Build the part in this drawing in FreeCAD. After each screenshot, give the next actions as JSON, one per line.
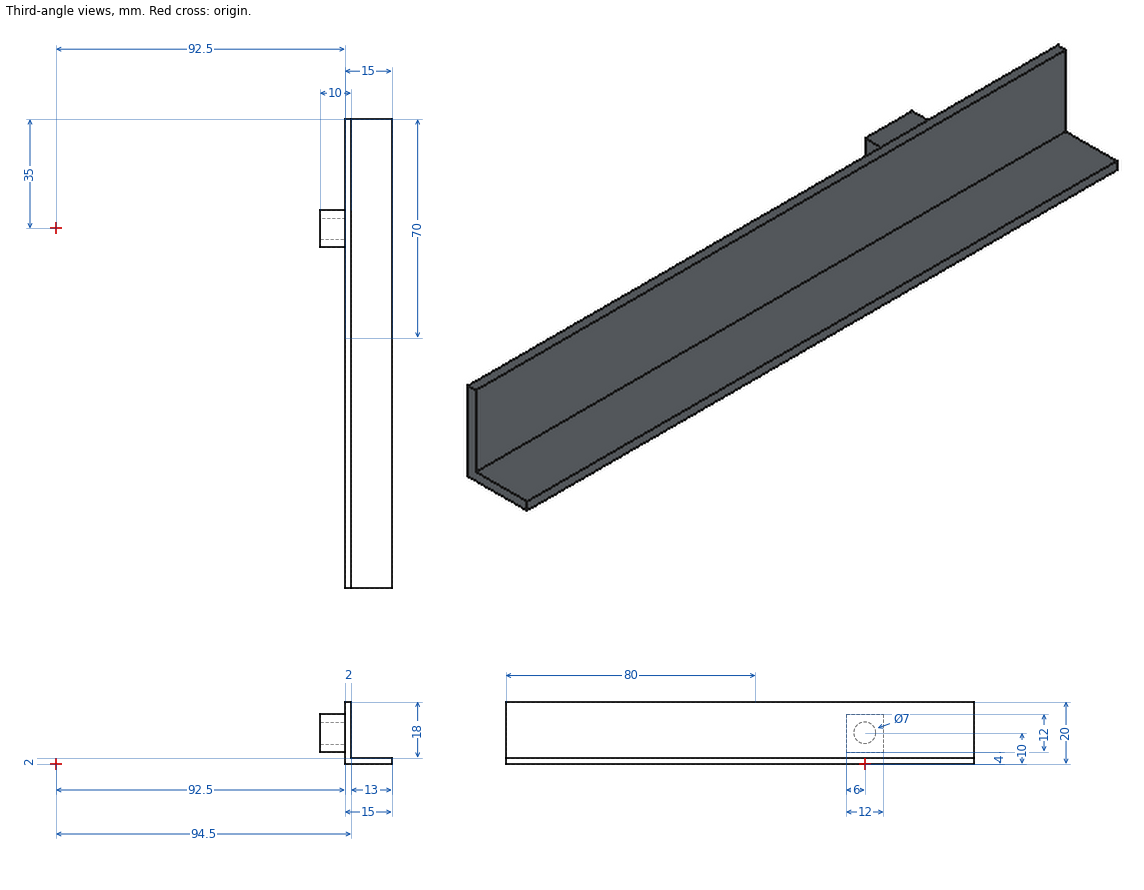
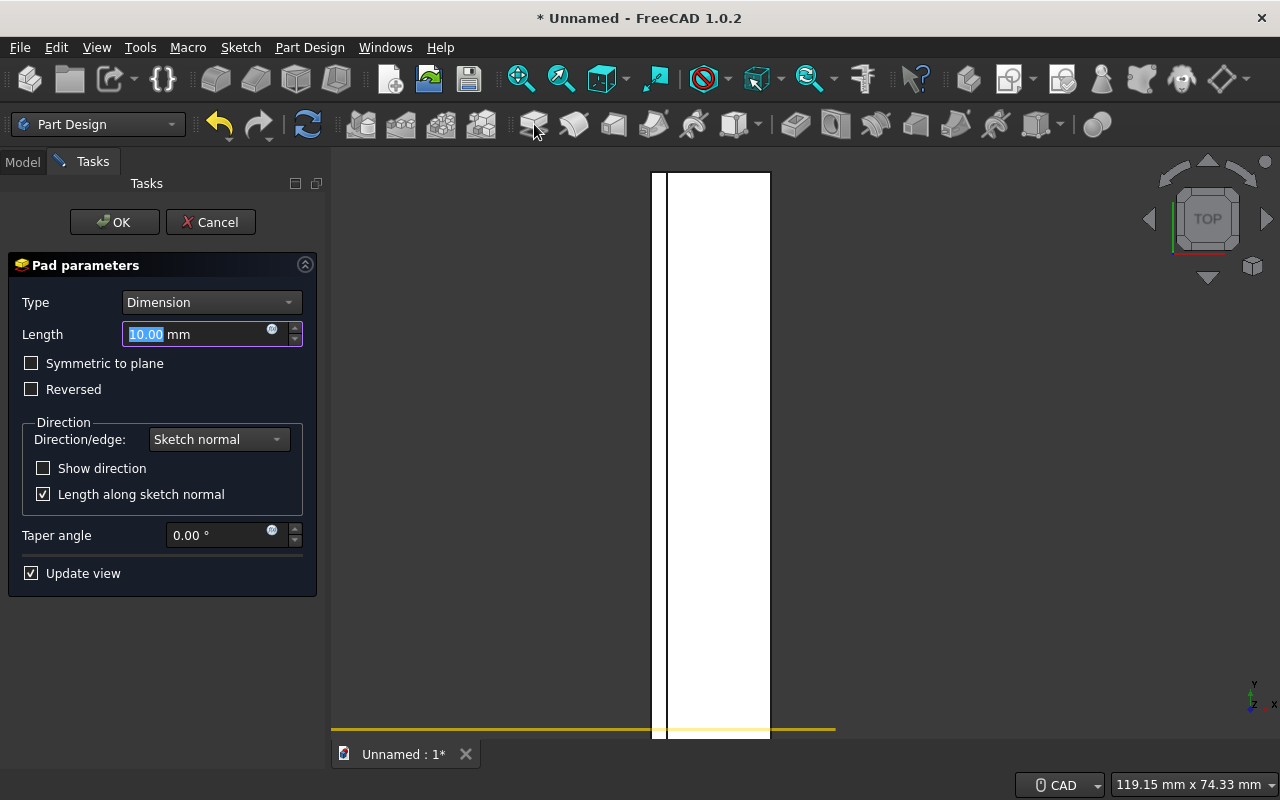
{"action": "type", "text": "80"}
{"action": "key", "text": "Tab"}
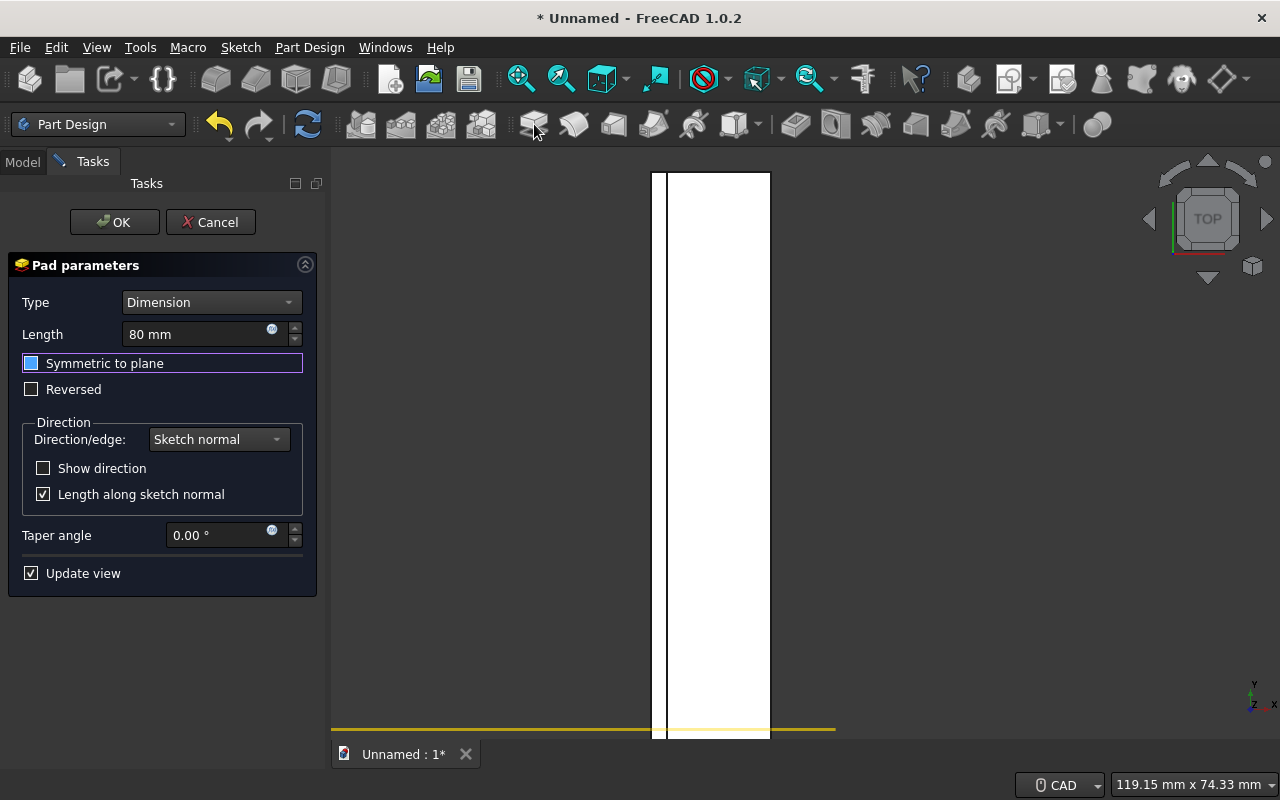
{"action": "left_click", "coordinate": [115, 222]}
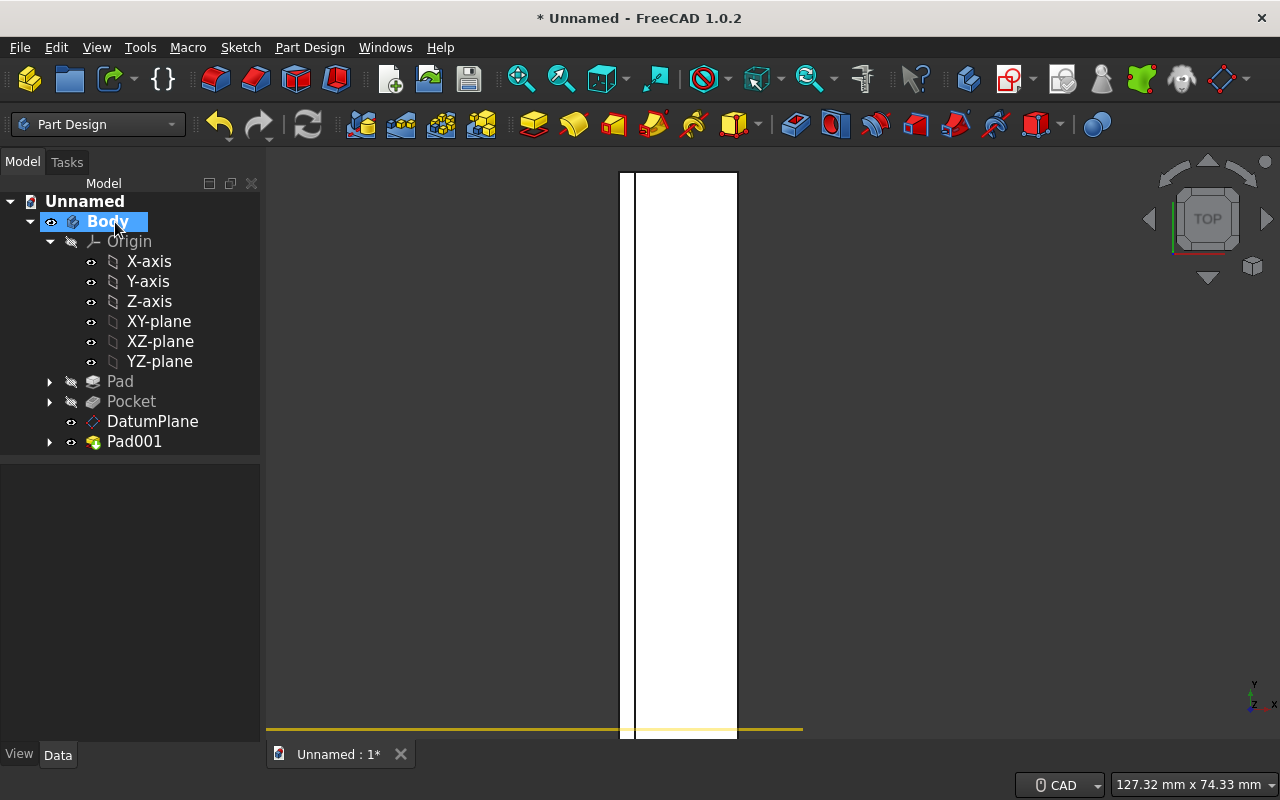
{"action": "left_click", "coordinate": [116, 422]}
{"action": "key", "text": "space"}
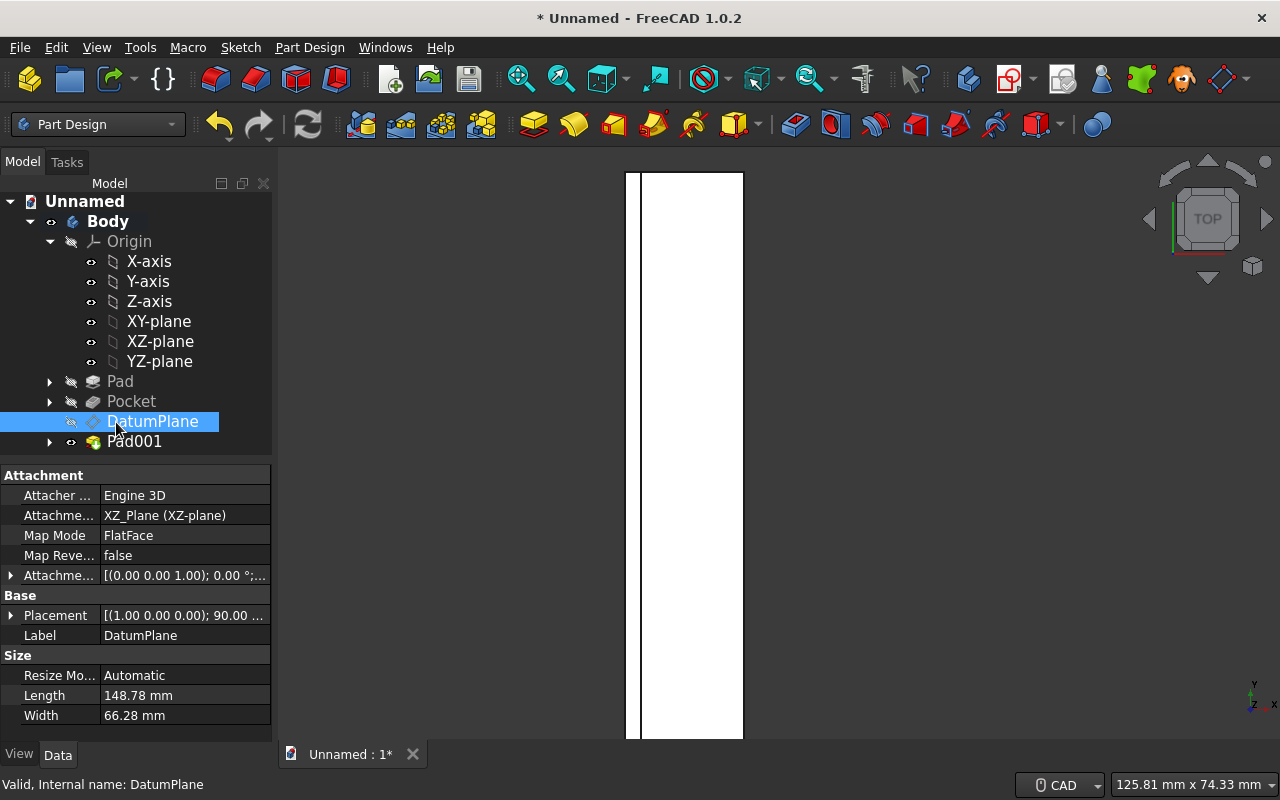
{"action": "left_click", "coordinate": [522, 80]}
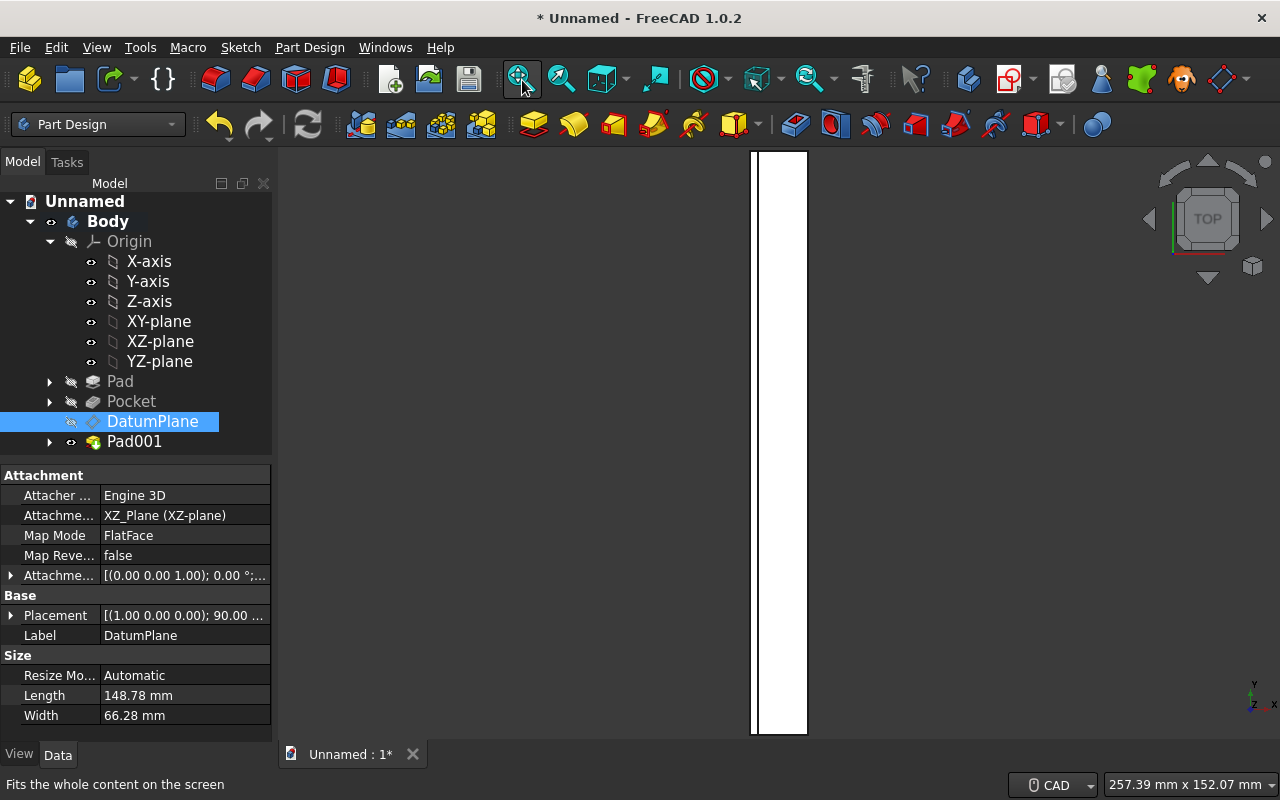
{"action": "key", "text": "0"}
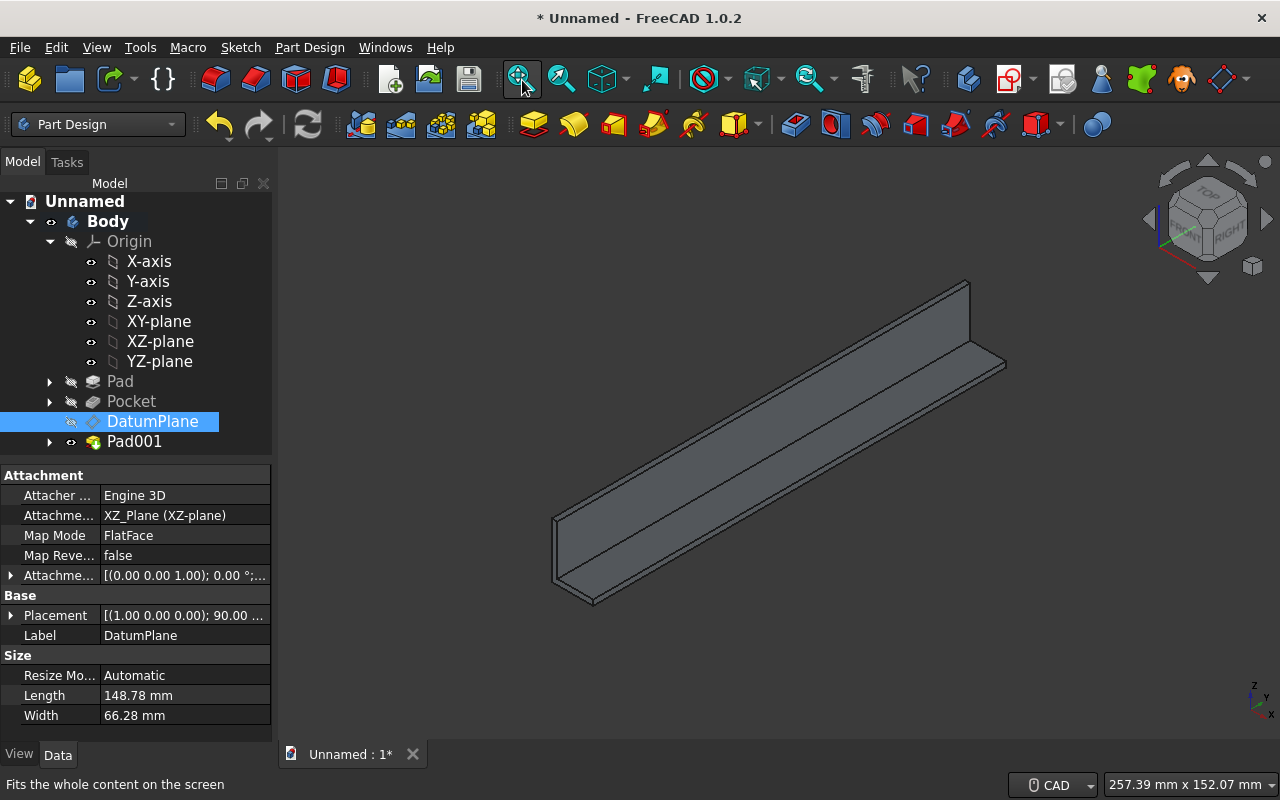
{"action": "left_click", "coordinate": [823, 396]}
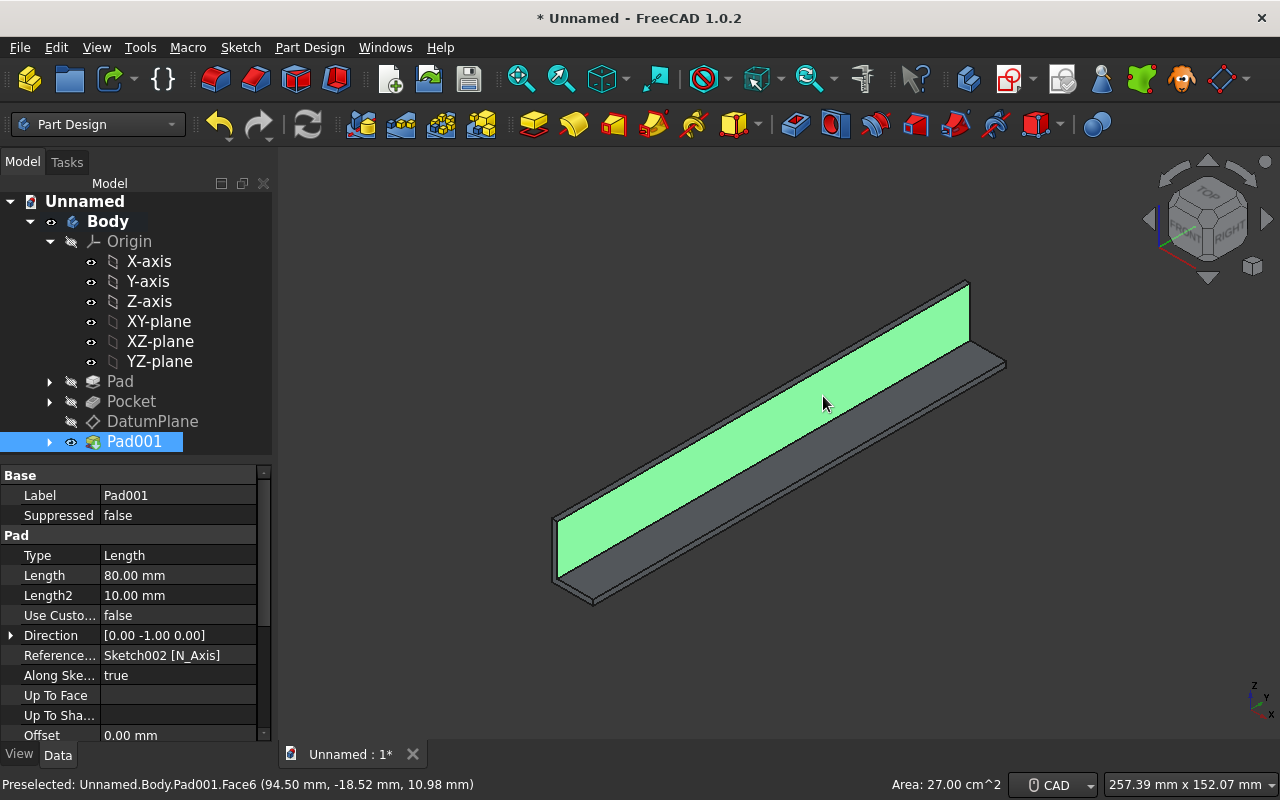
{"action": "left_click", "coordinate": [1010, 80]}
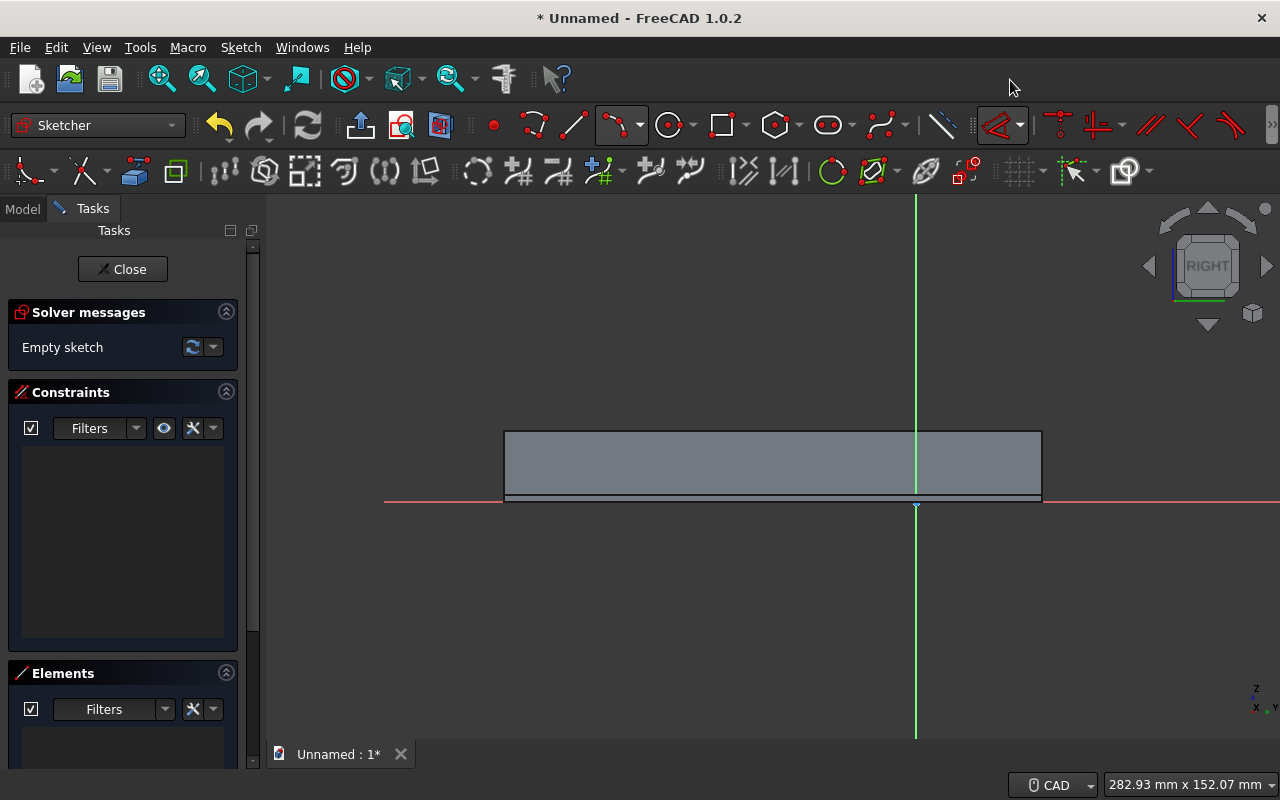
{"action": "left_click", "coordinate": [442, 126]}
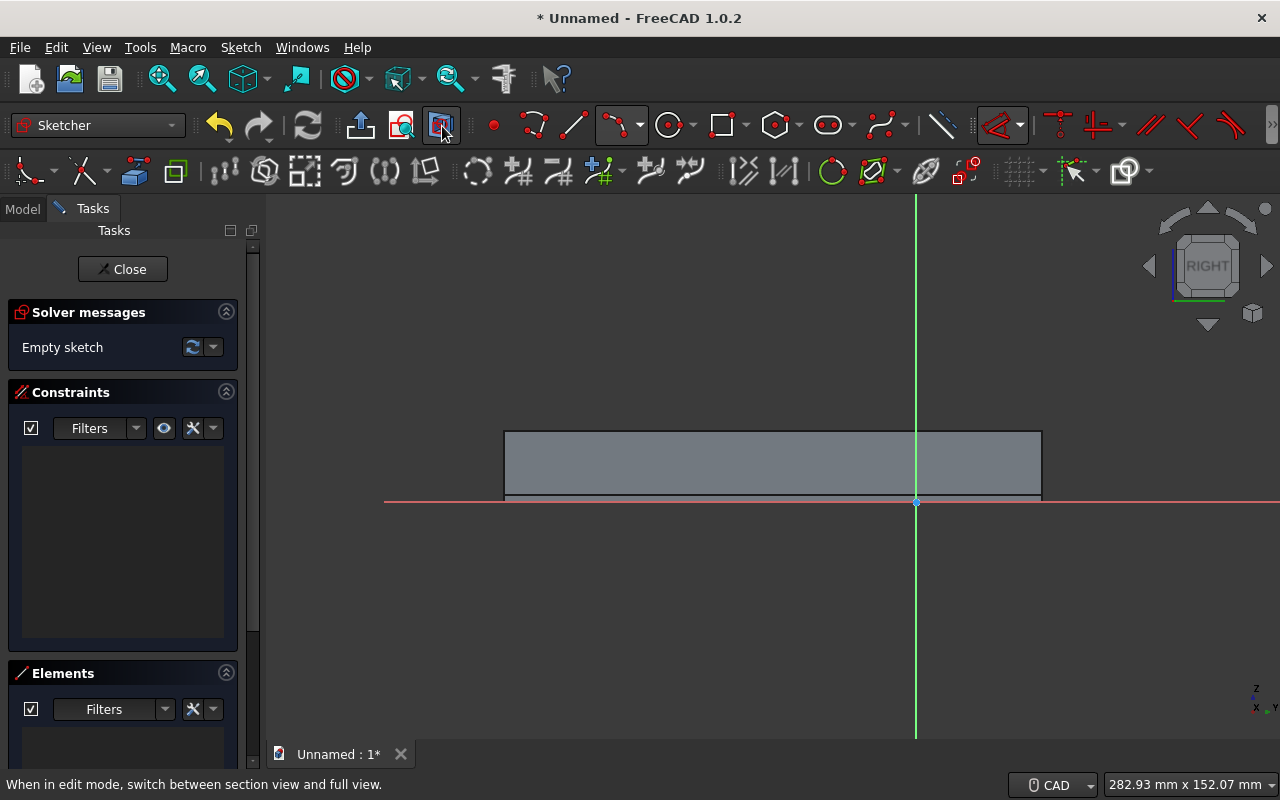
{"action": "scroll", "coordinate": [958, 475], "scroll_direction": "up", "scroll_amount": 9}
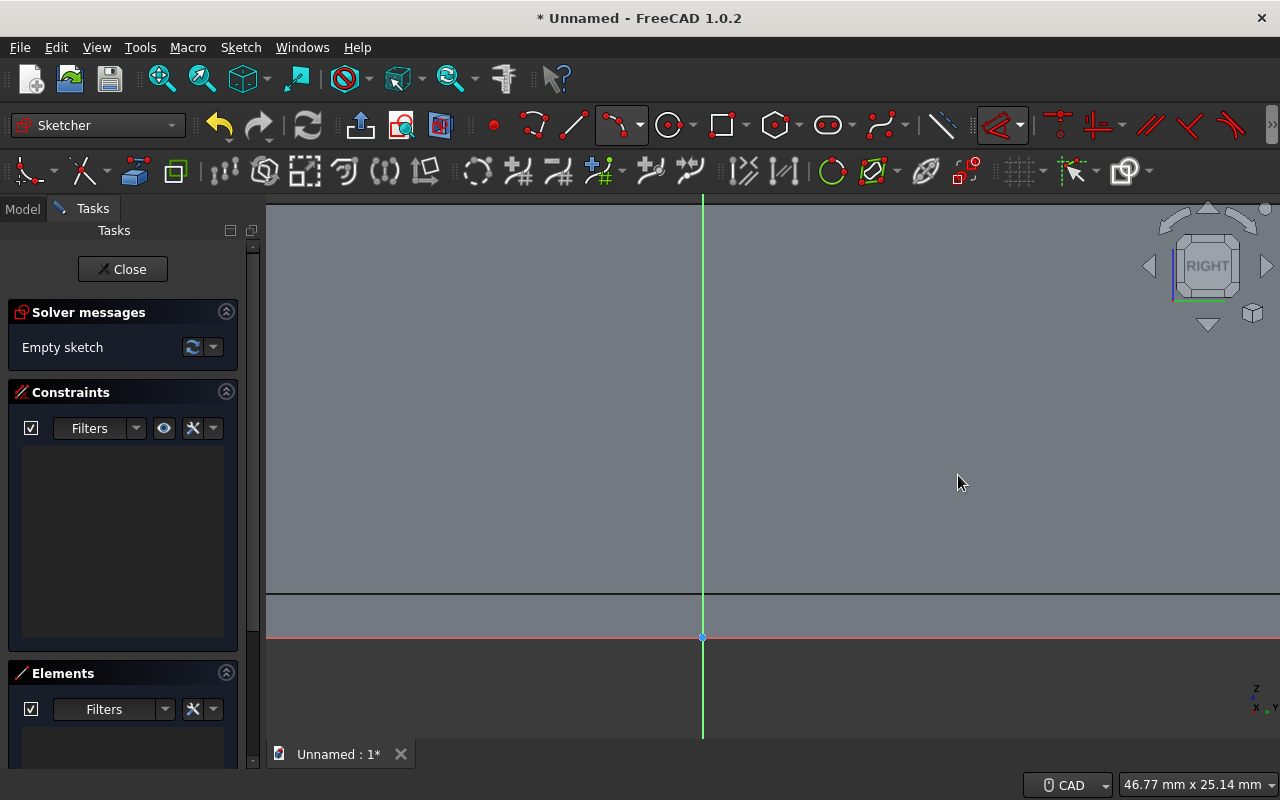
{"action": "left_click", "coordinate": [722, 126]}